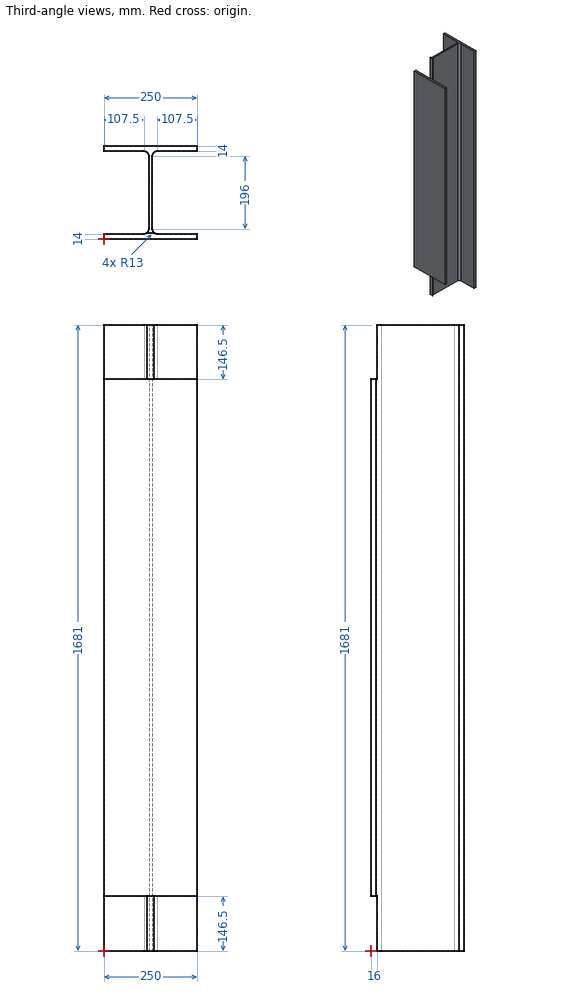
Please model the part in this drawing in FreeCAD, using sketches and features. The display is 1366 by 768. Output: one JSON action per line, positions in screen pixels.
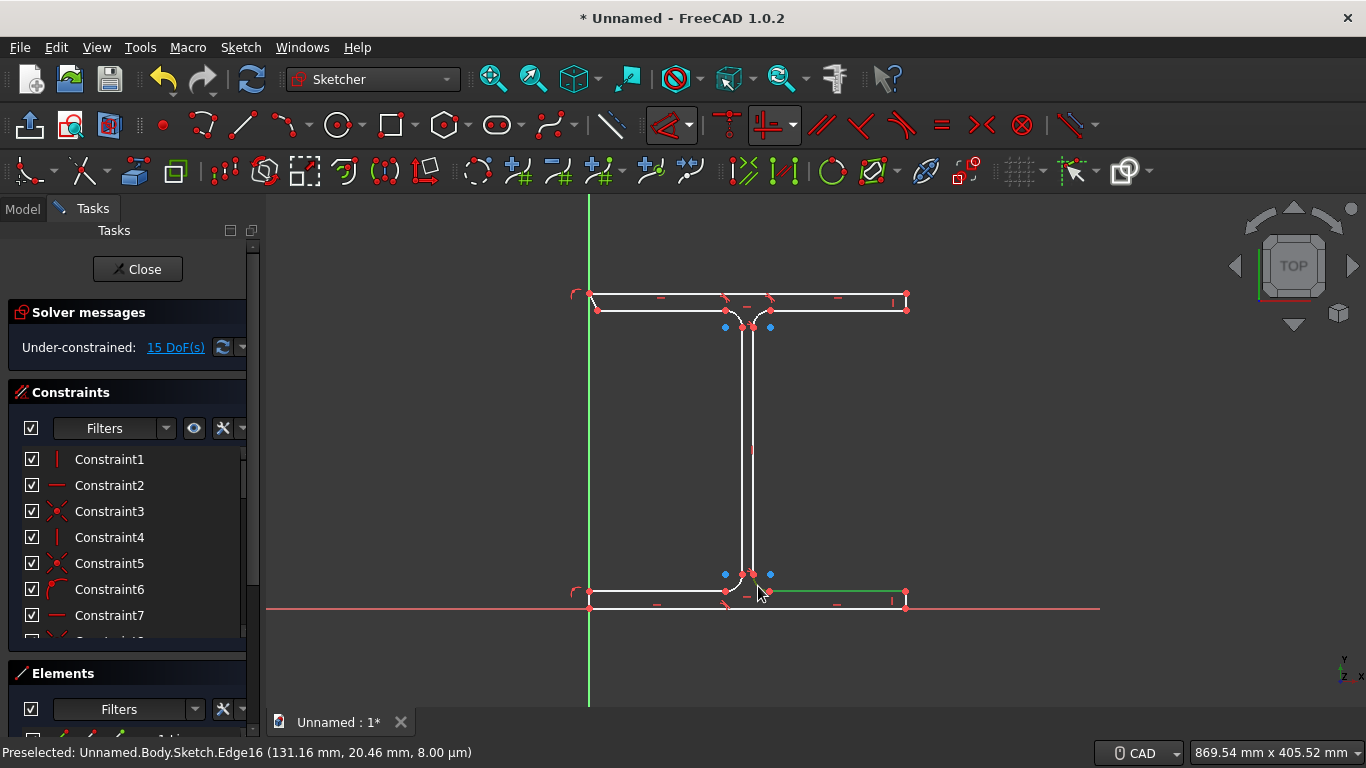
{"action": "left_click", "coordinate": [902, 126]}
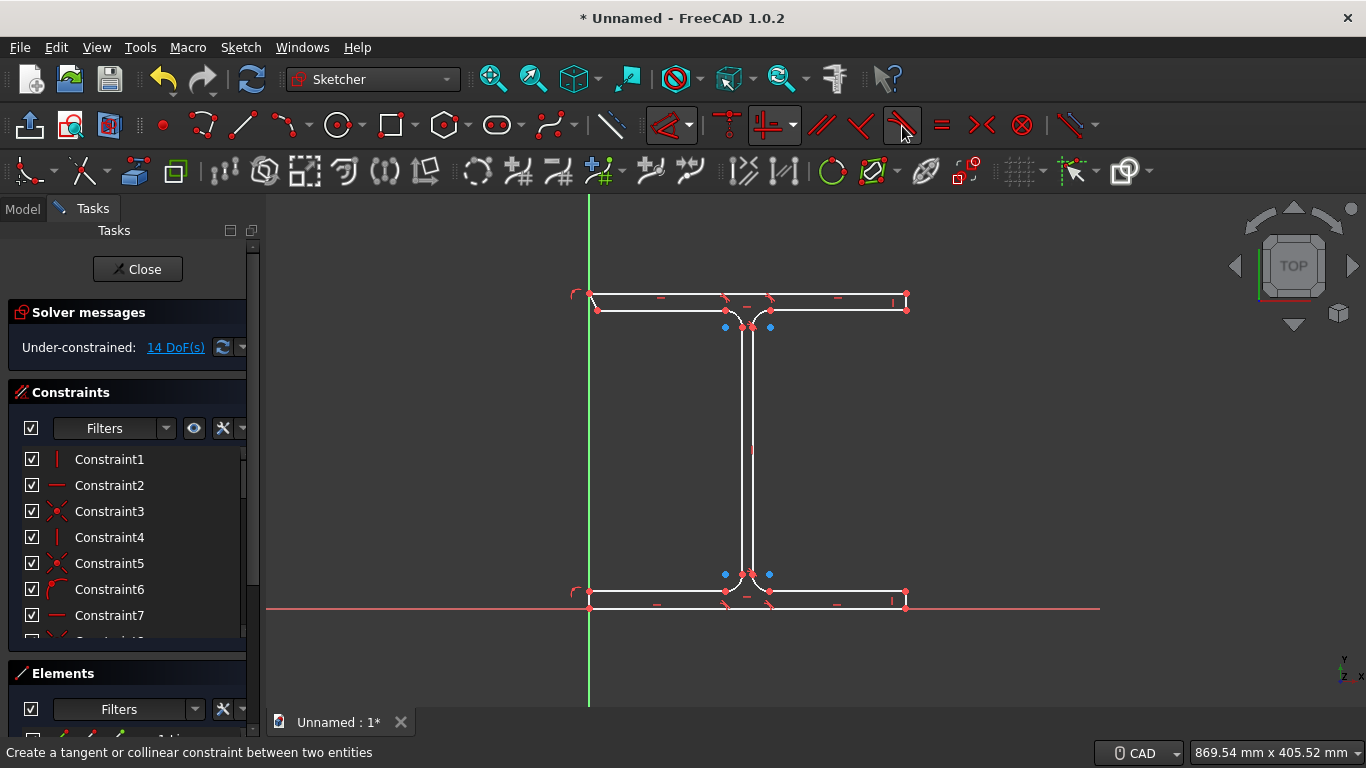
{"action": "scroll", "coordinate": [593, 301], "scroll_direction": "up", "scroll_amount": 4}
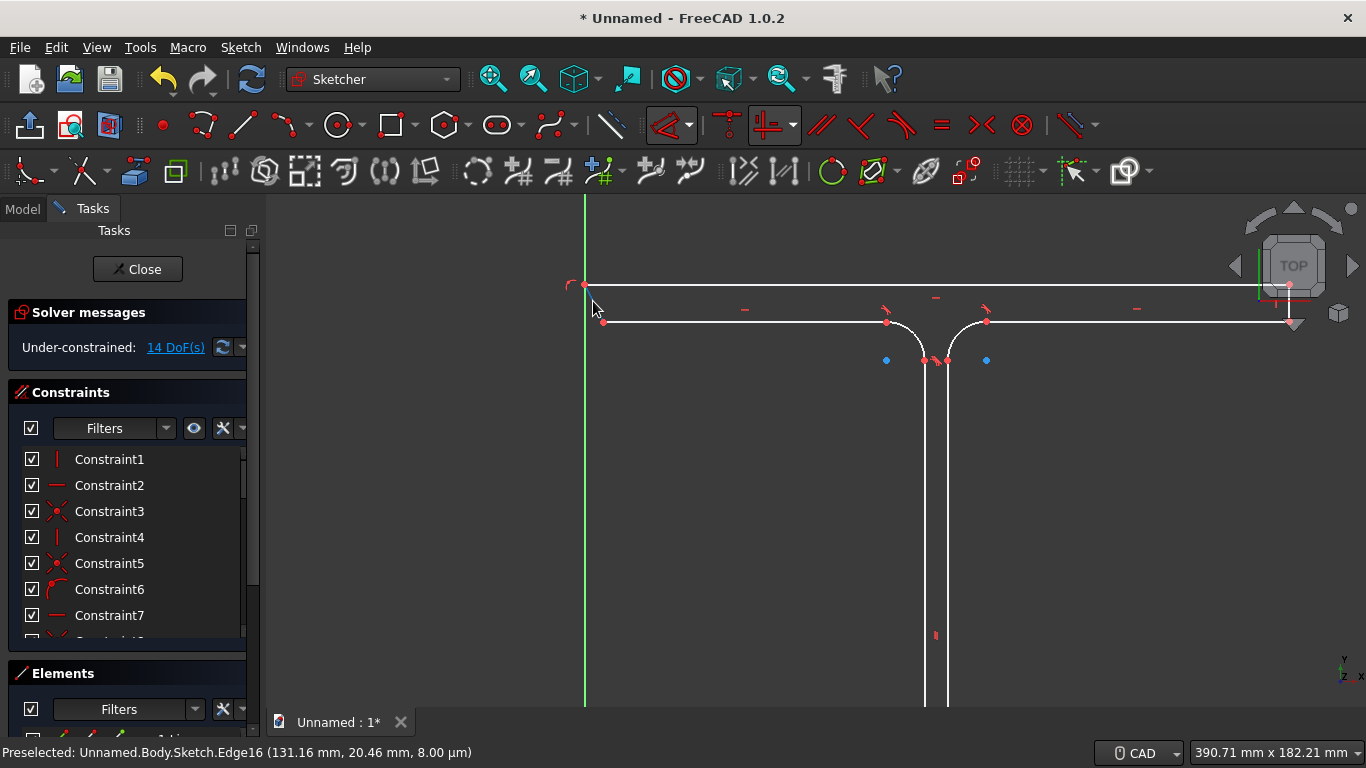
{"action": "left_click", "coordinate": [592, 300]}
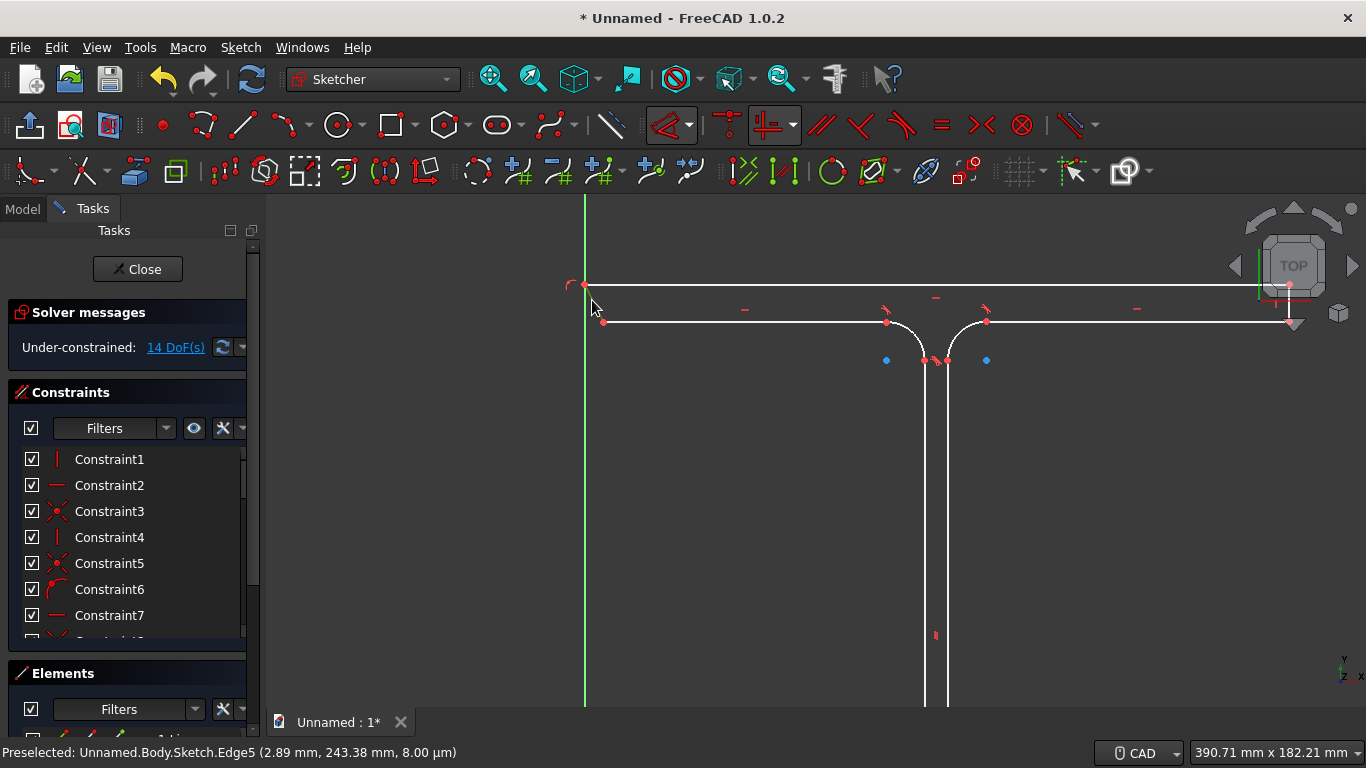
{"action": "left_click", "coordinate": [796, 126]}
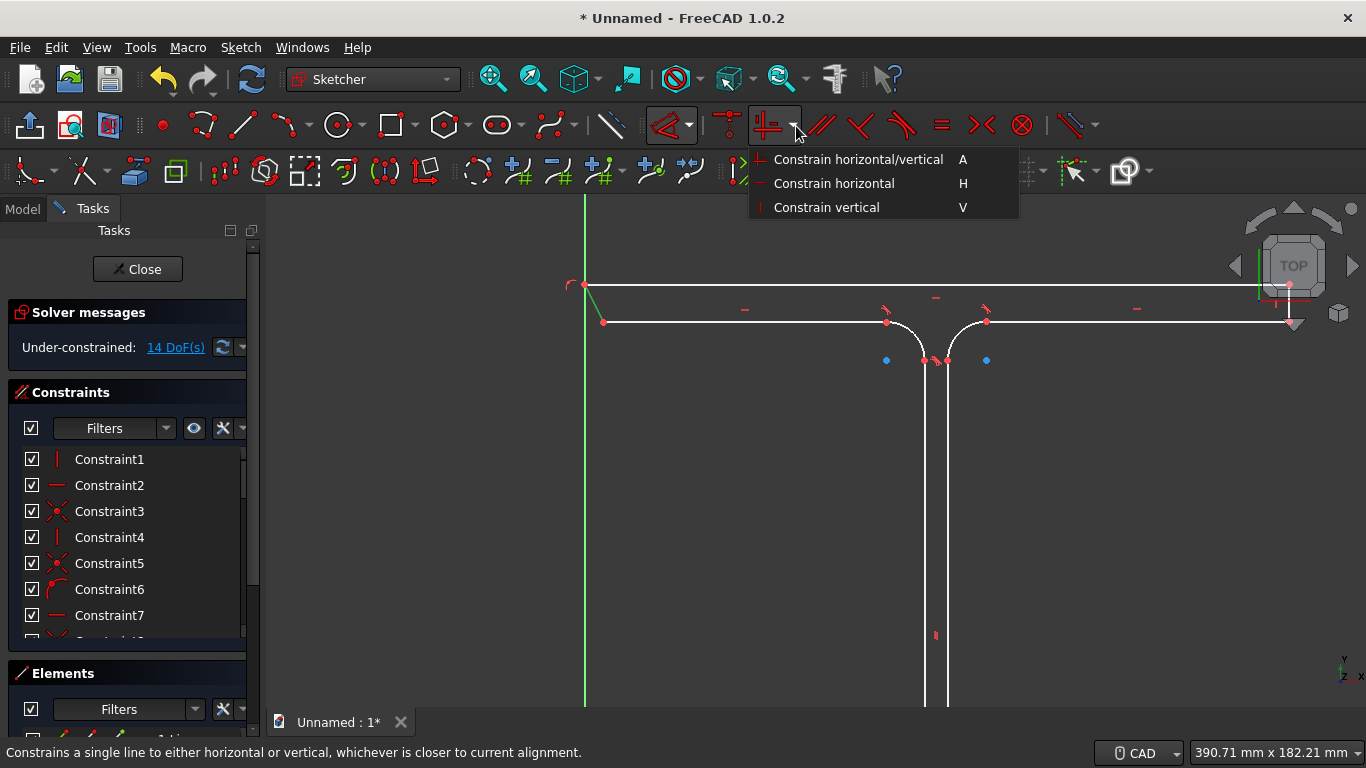
{"action": "left_click", "coordinate": [884, 207]}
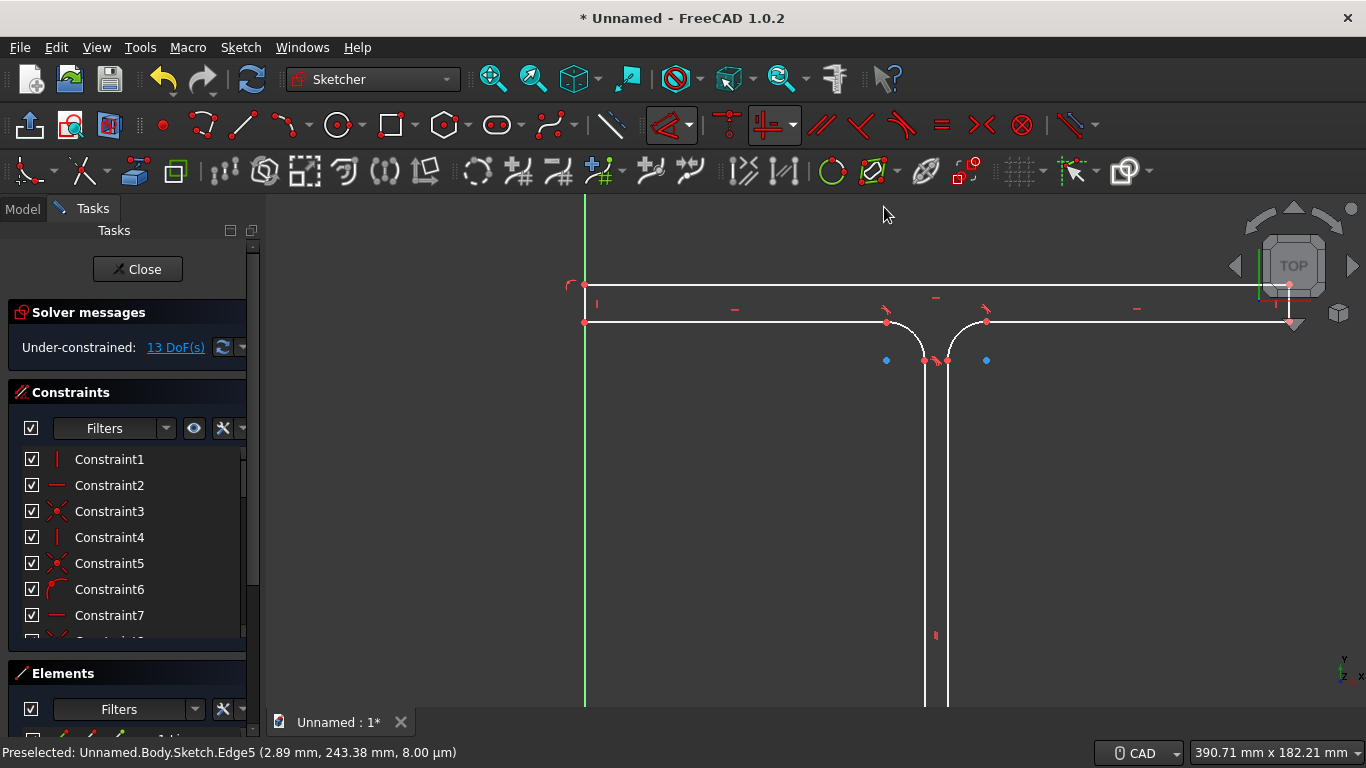
{"action": "left_click", "coordinate": [969, 326]}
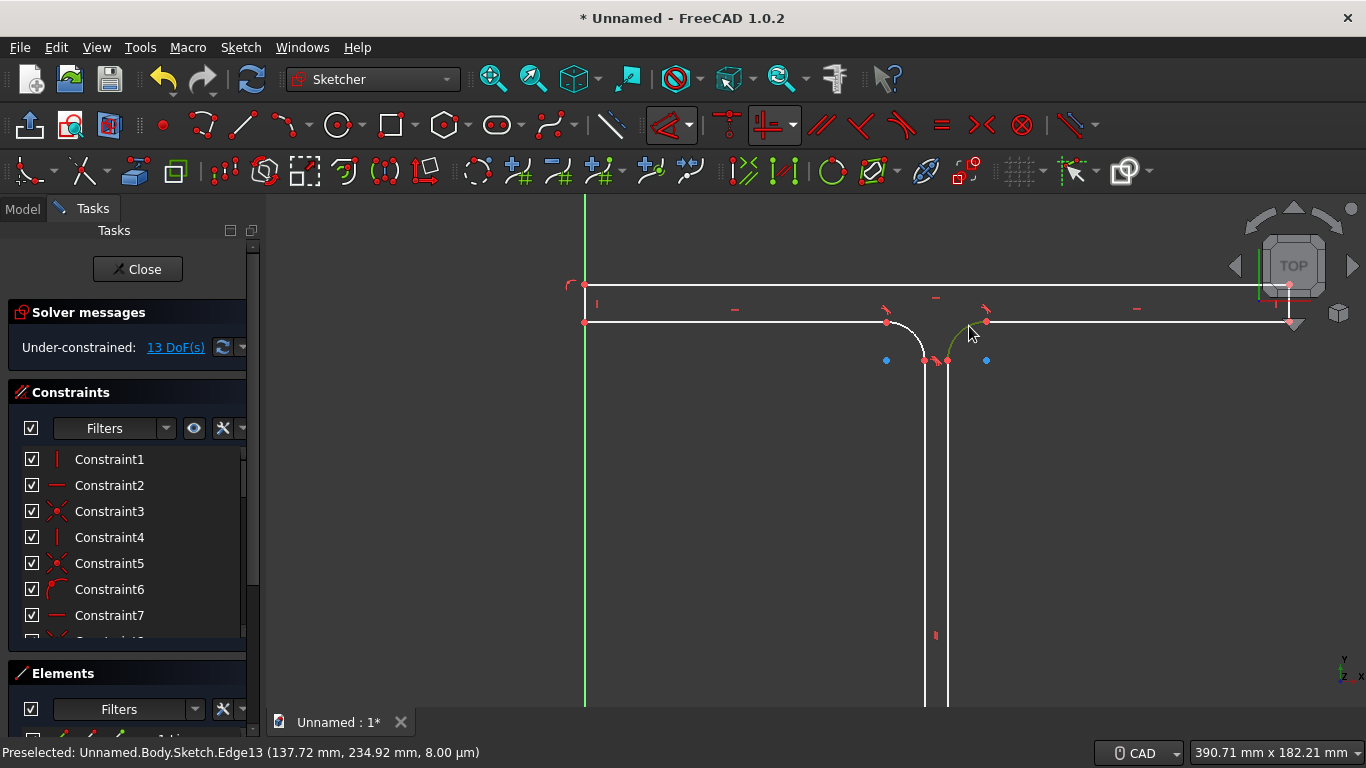
{"action": "left_click", "coordinate": [920, 343]}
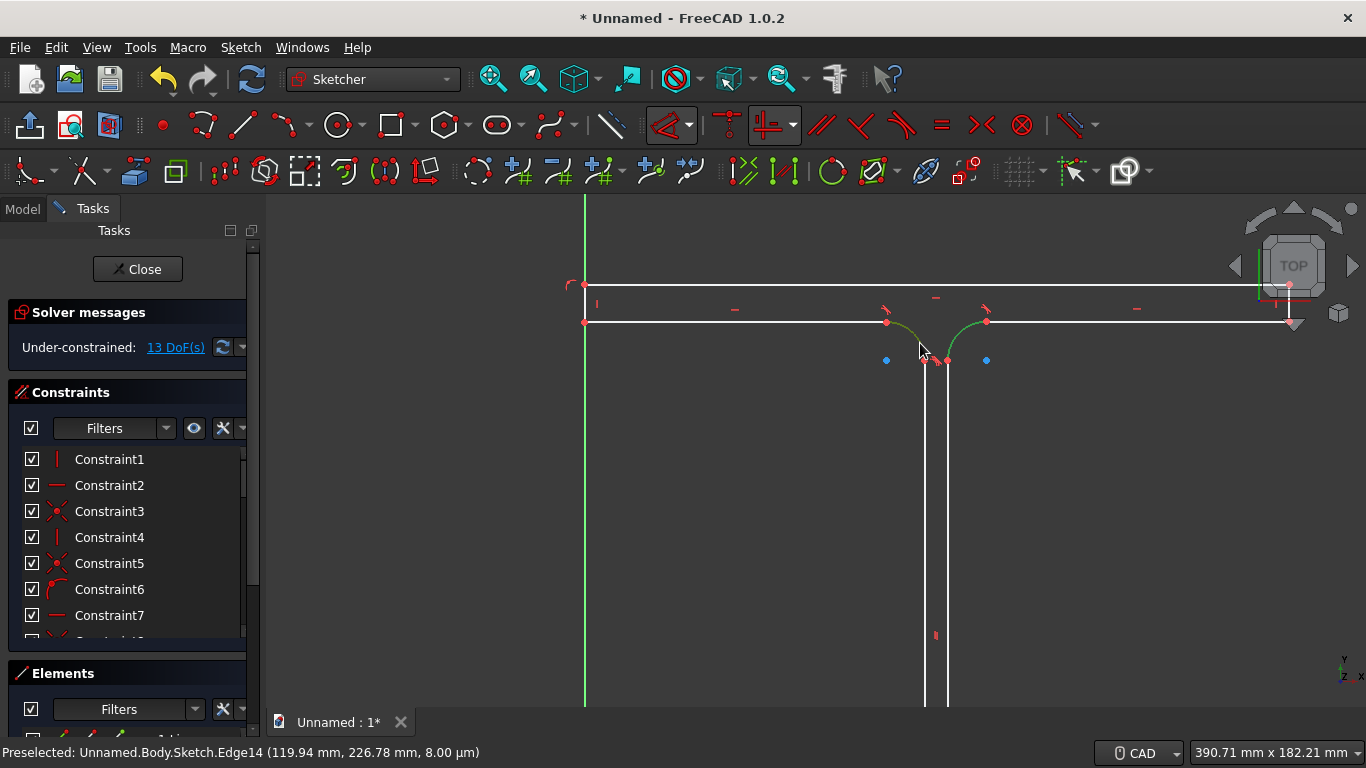
{"action": "scroll", "coordinate": [593, 301], "scroll_direction": "down", "scroll_amount": 4}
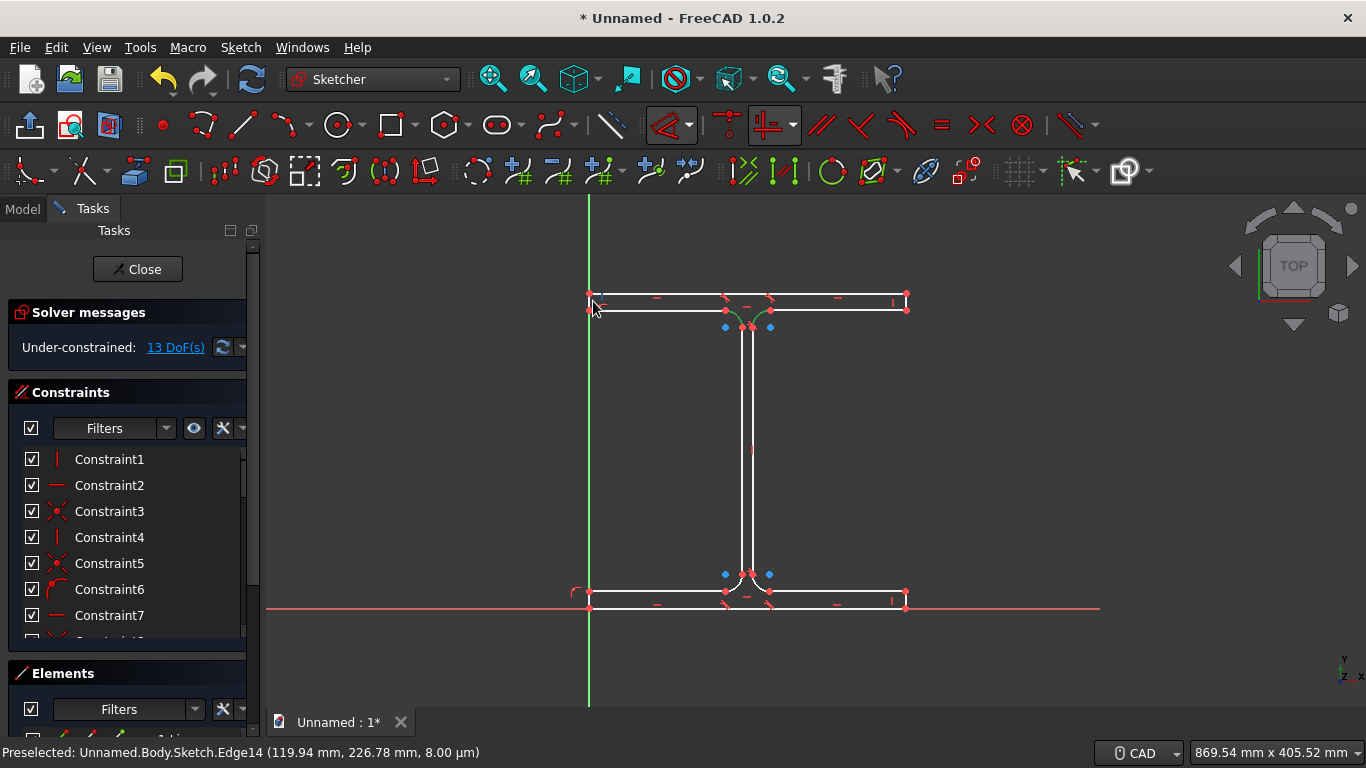
{"action": "scroll", "coordinate": [733, 590], "scroll_direction": "up", "scroll_amount": 3}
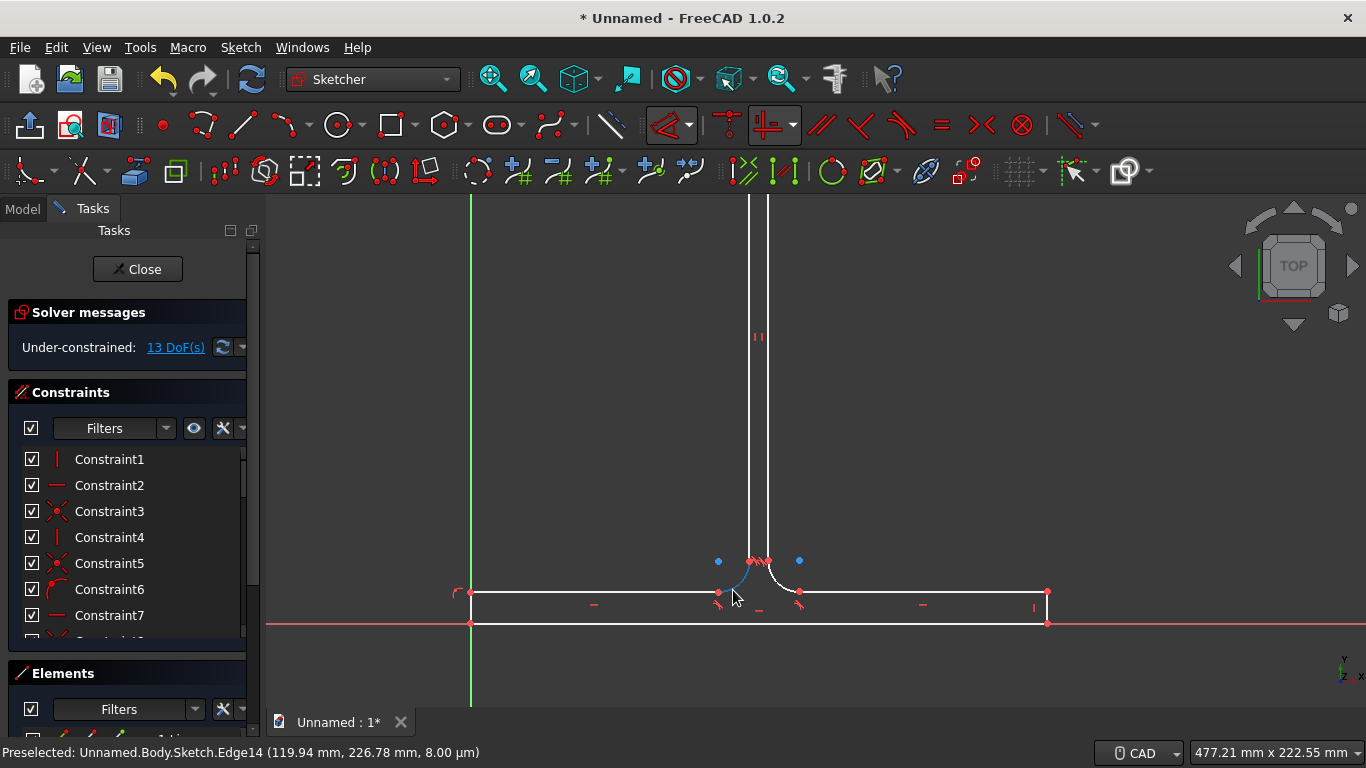
{"action": "left_click", "coordinate": [733, 589]}